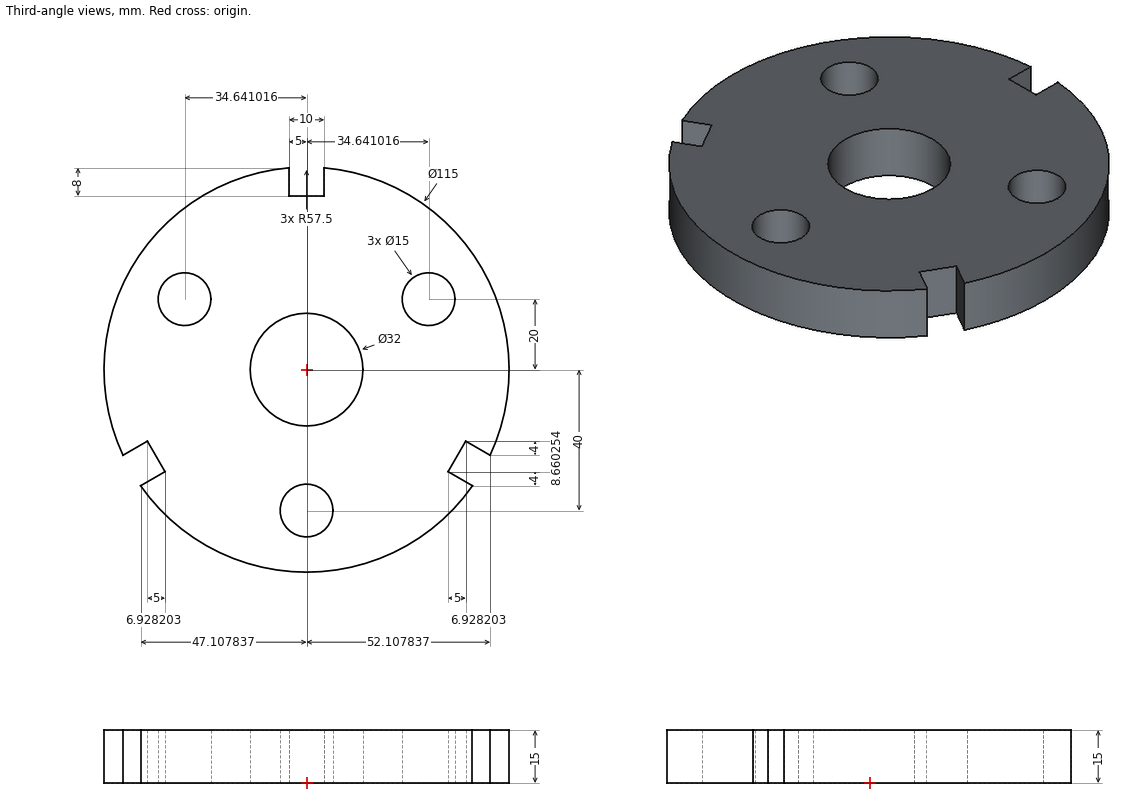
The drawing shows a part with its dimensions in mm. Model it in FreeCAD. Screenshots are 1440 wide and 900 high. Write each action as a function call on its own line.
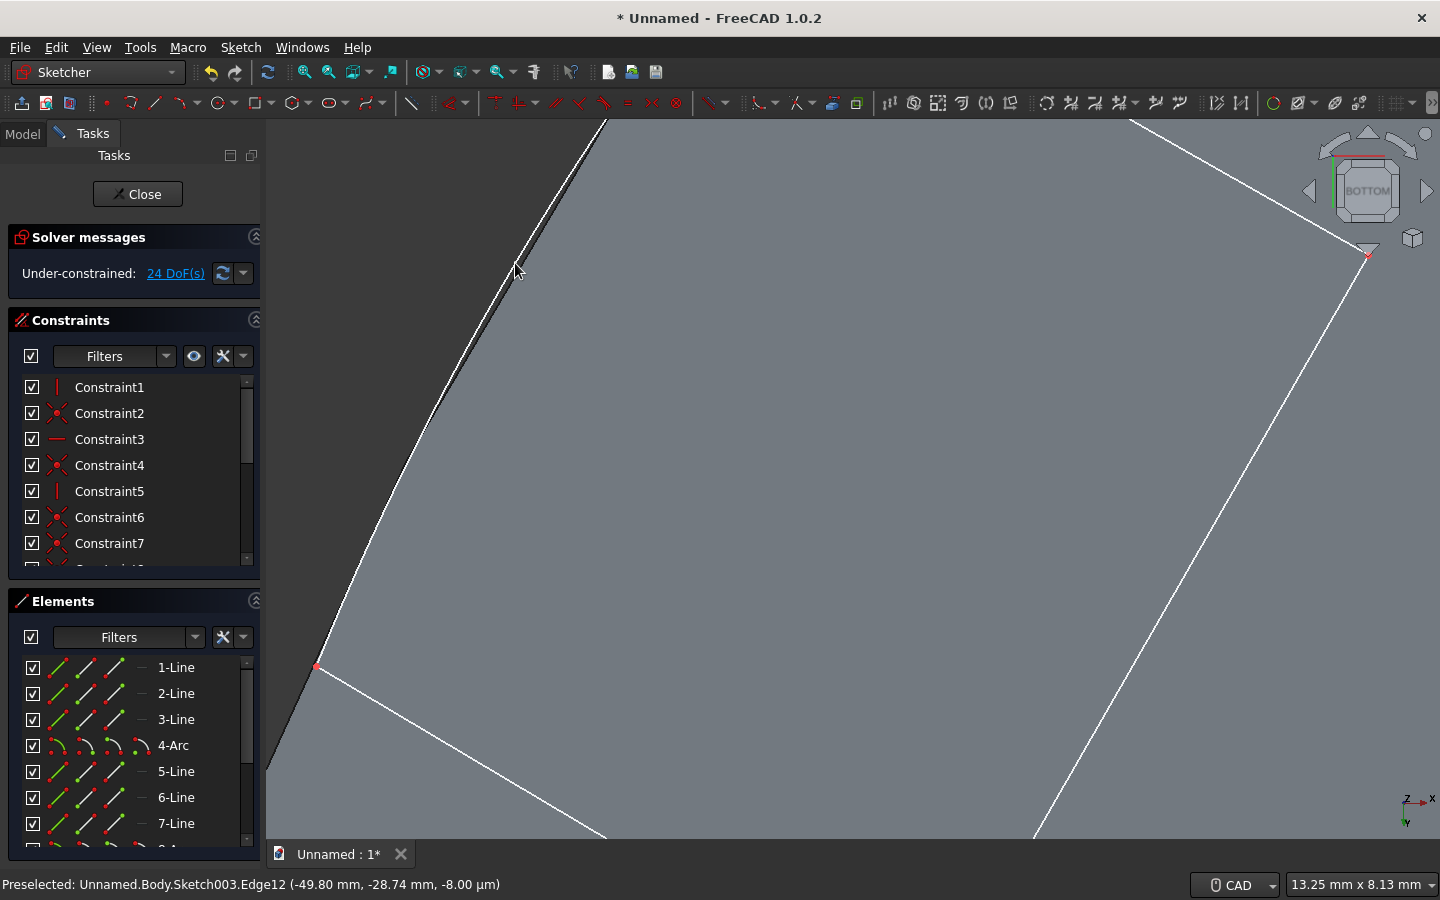
scroll(516, 258, down, 14)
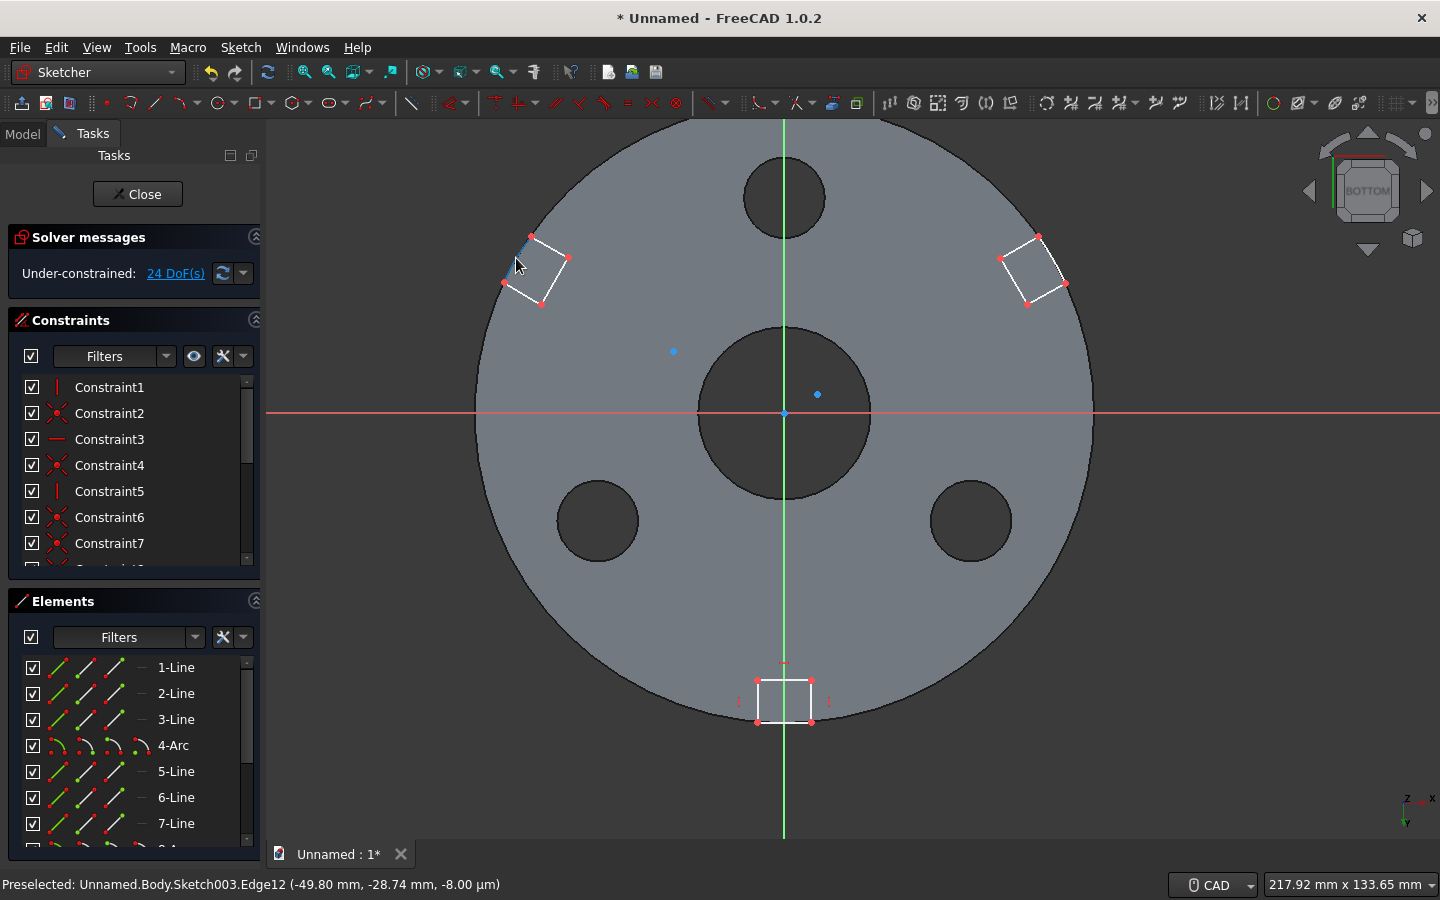
scroll(774, 723, up, 2)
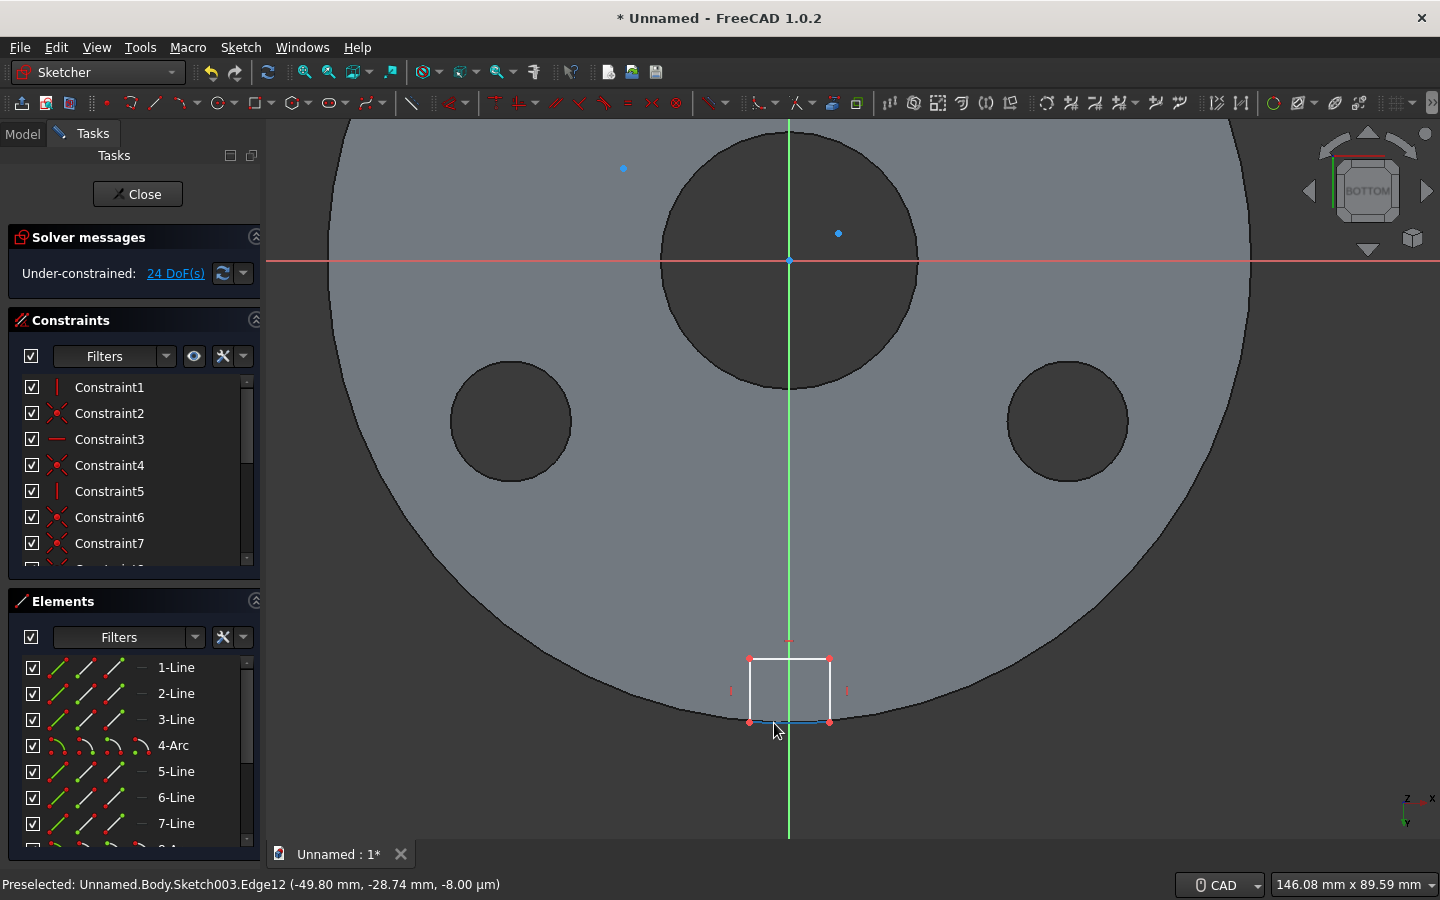
click(774, 723)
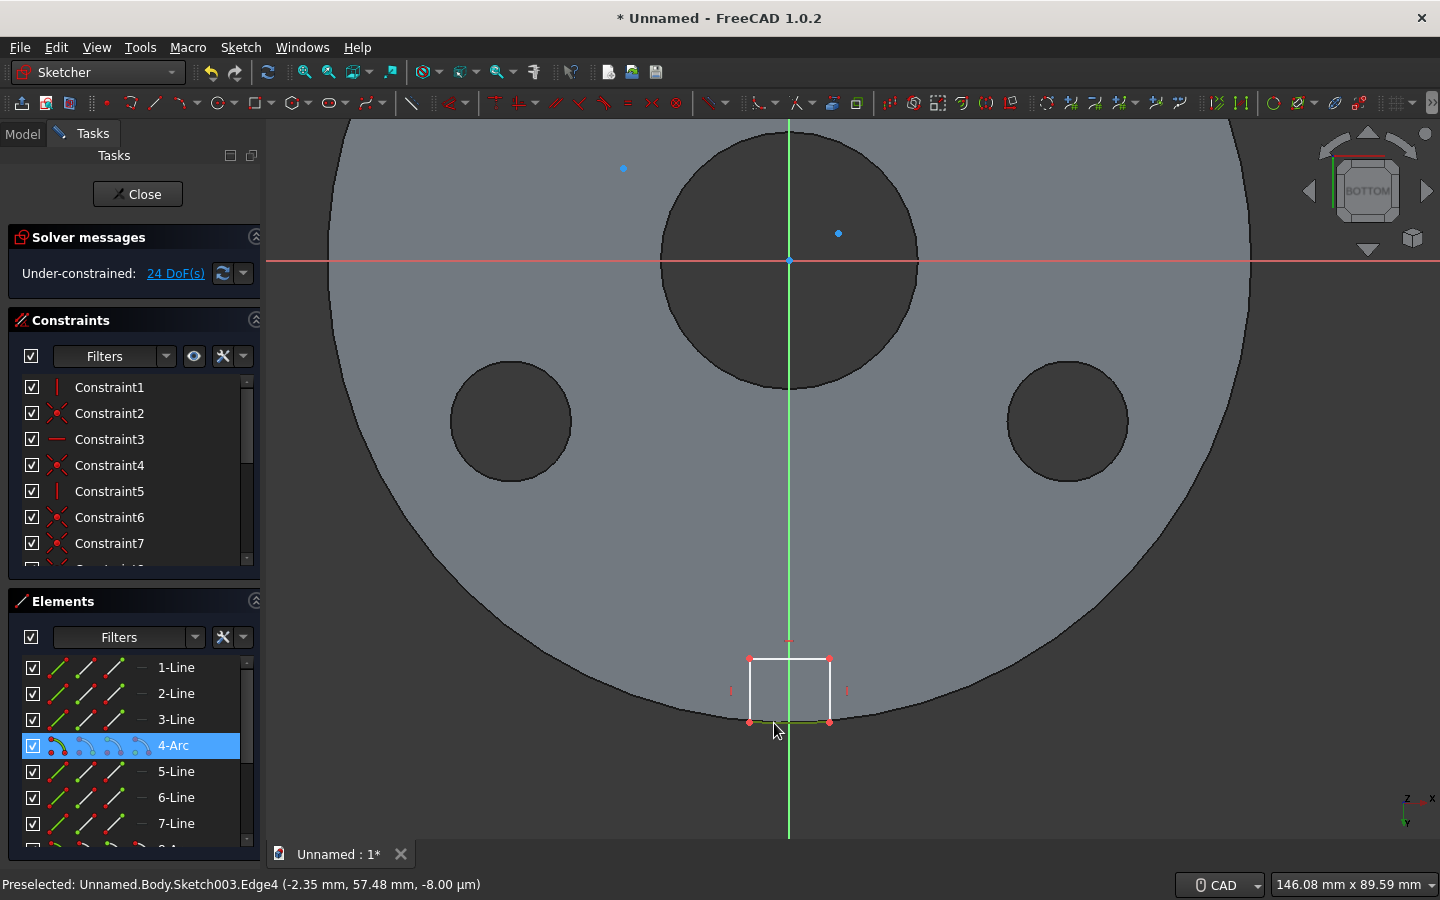
scroll(775, 723, down, 2)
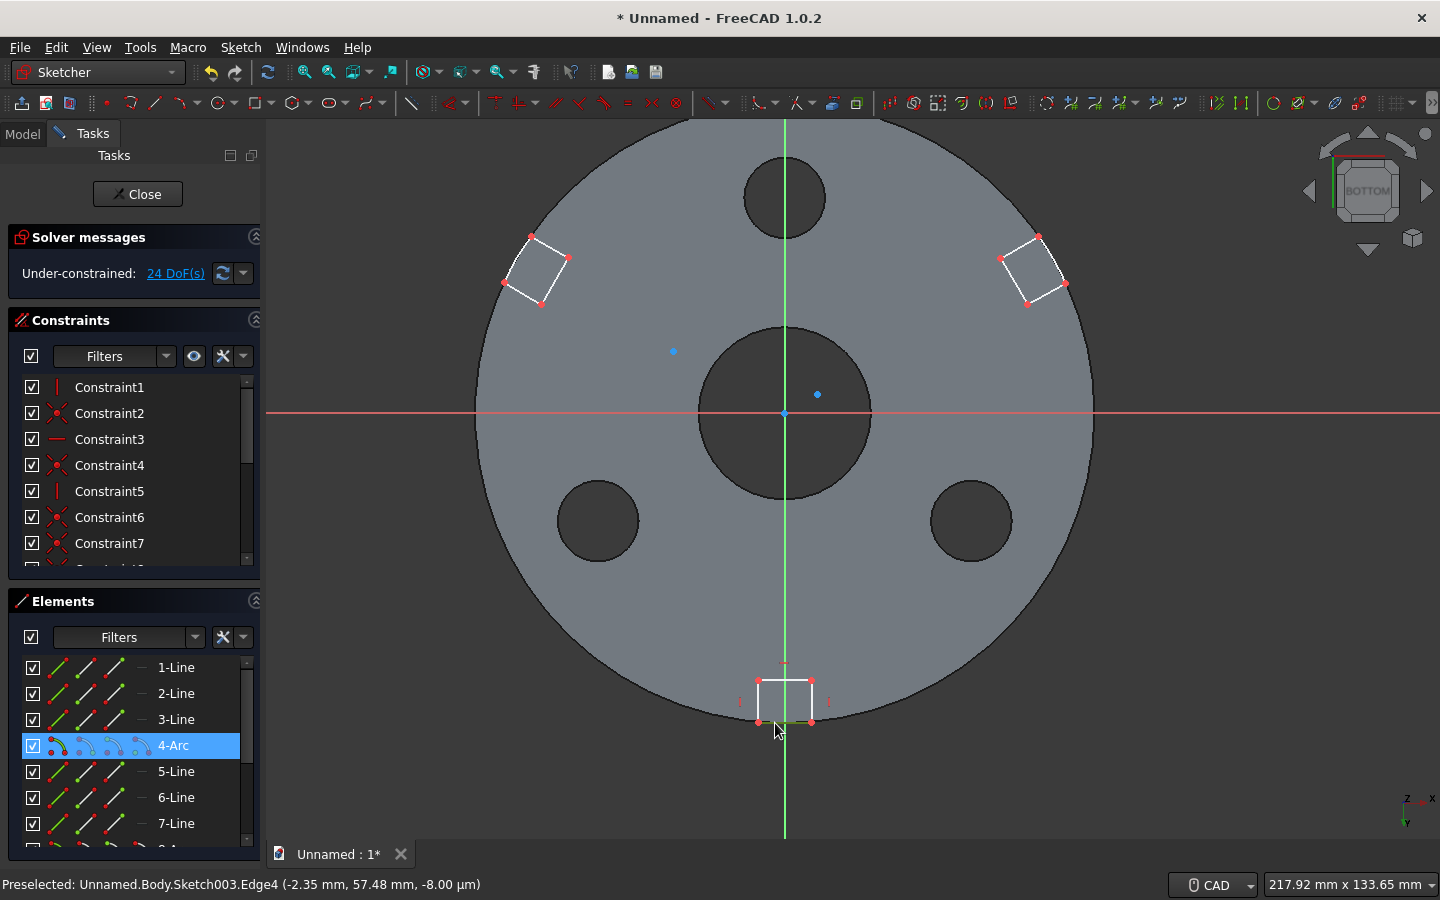
click(1059, 269)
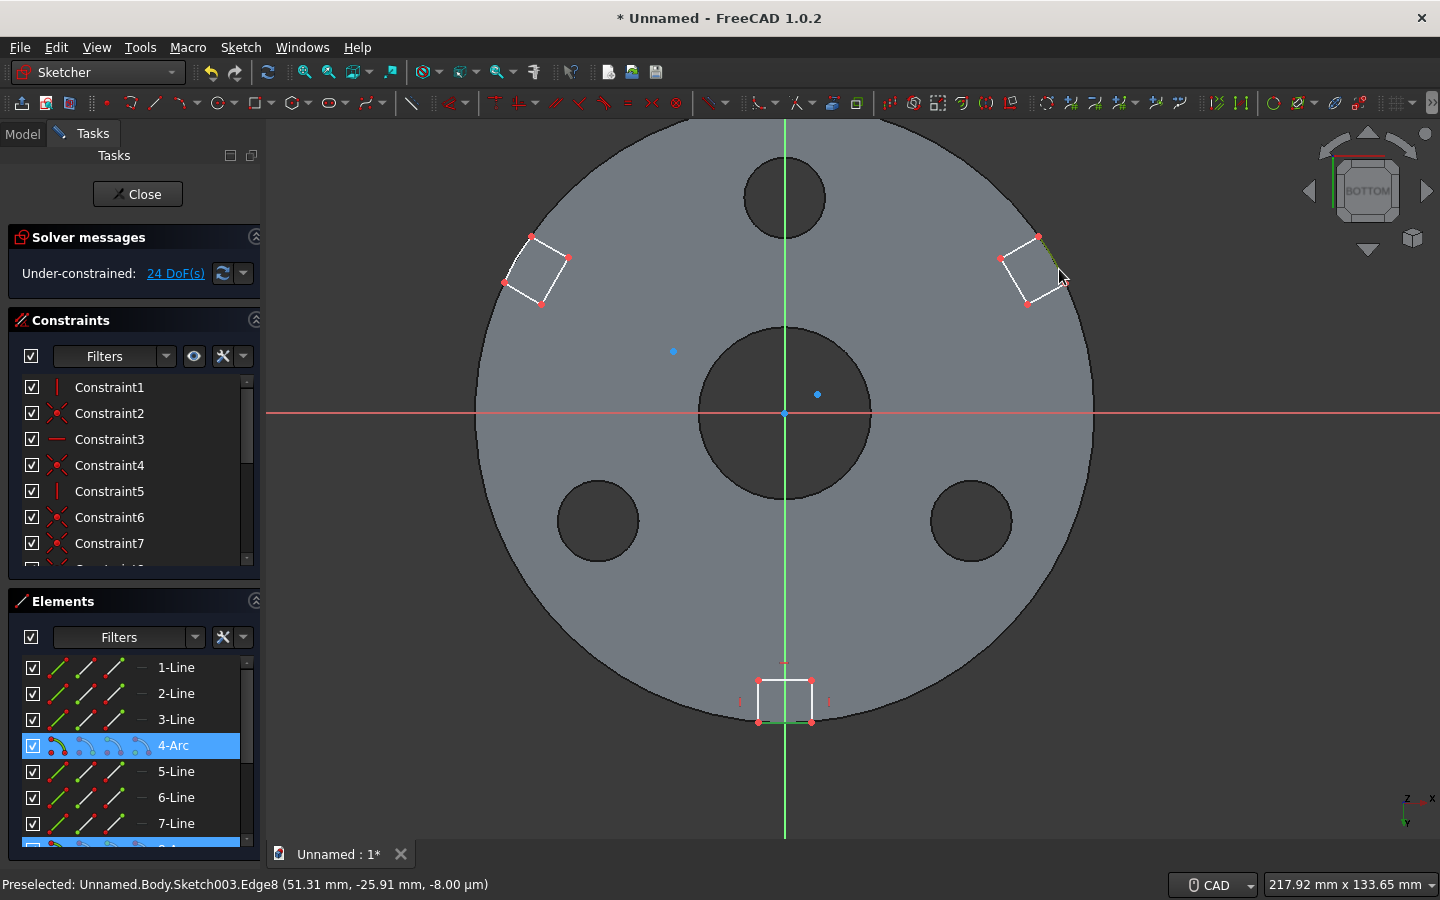
click(496, 104)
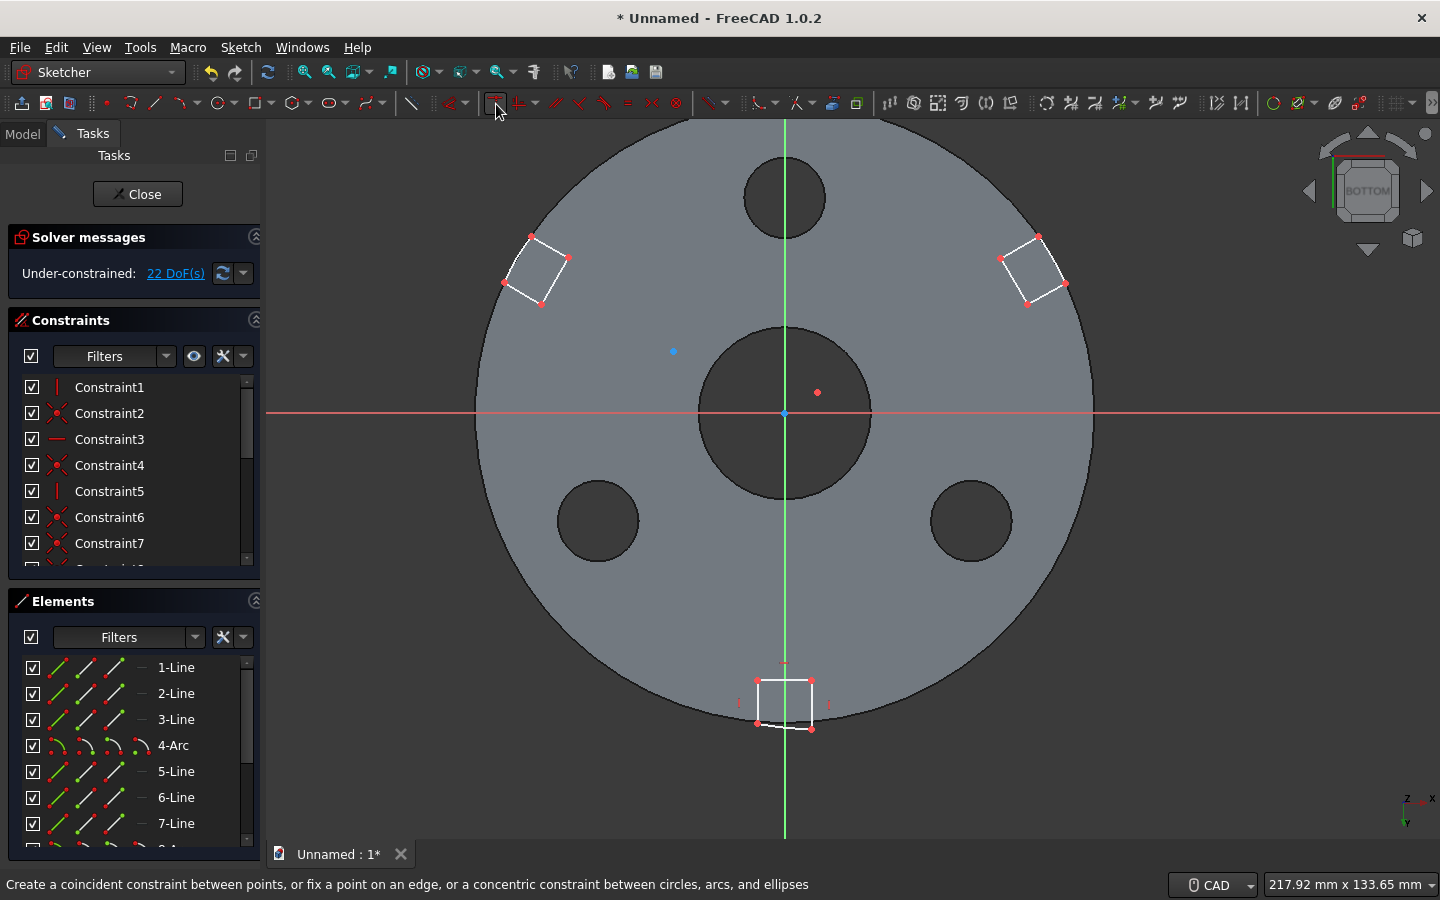
scroll(774, 726, up, 2)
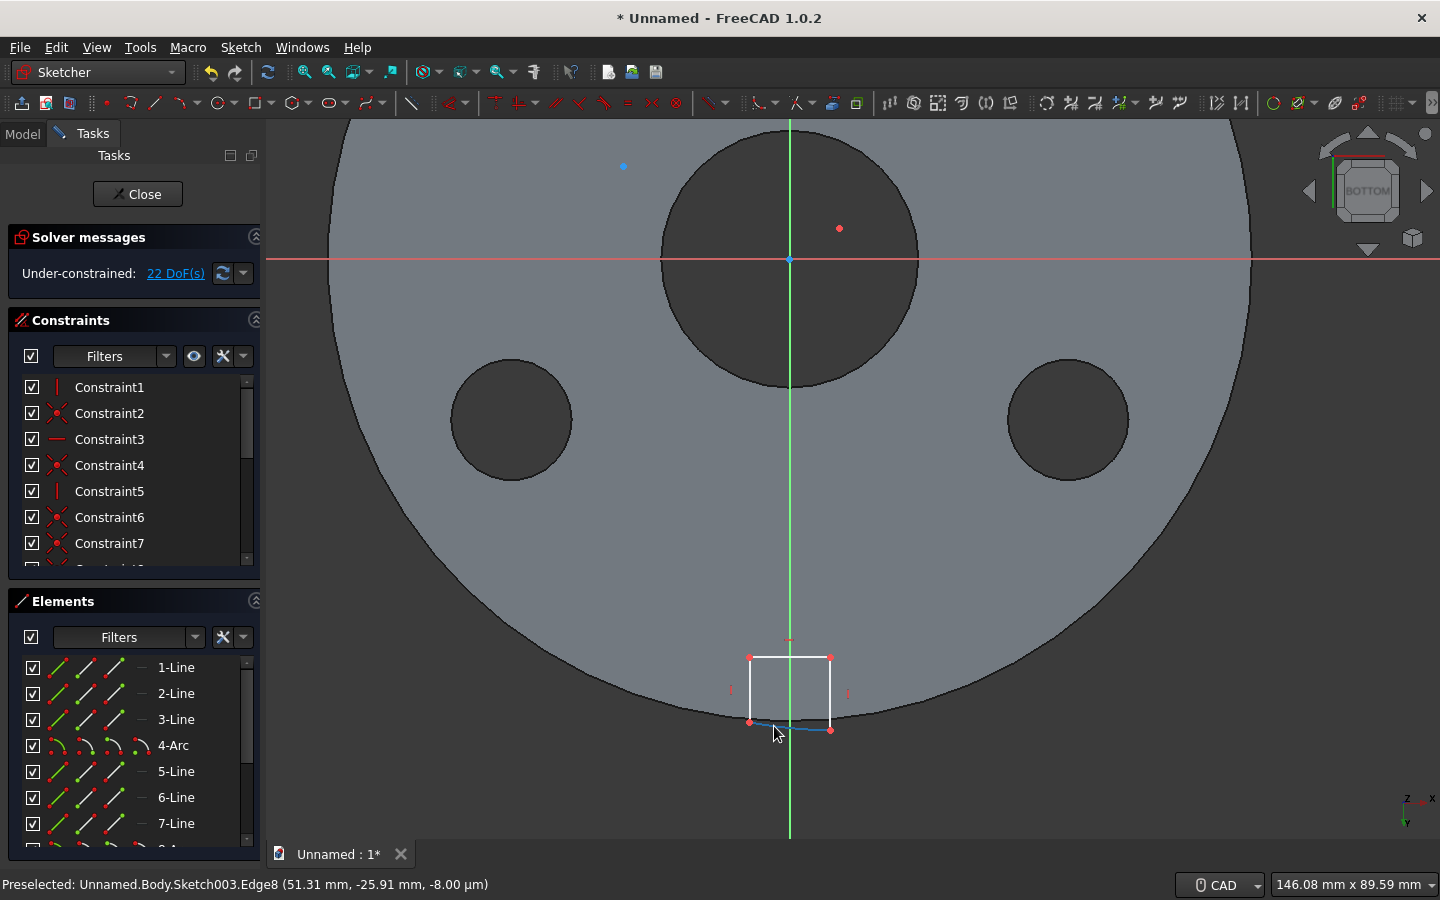
click(774, 726)